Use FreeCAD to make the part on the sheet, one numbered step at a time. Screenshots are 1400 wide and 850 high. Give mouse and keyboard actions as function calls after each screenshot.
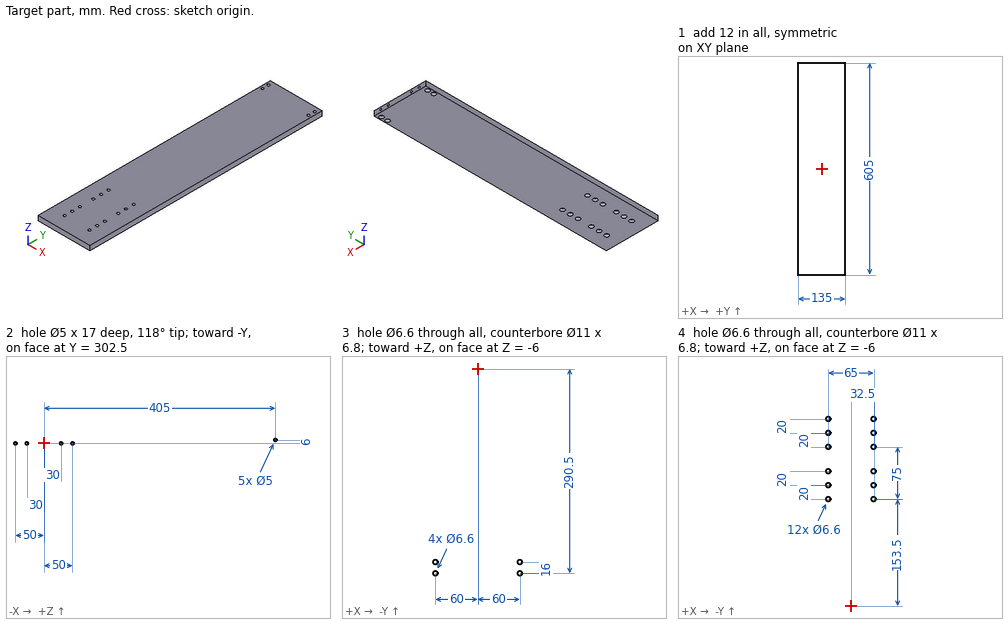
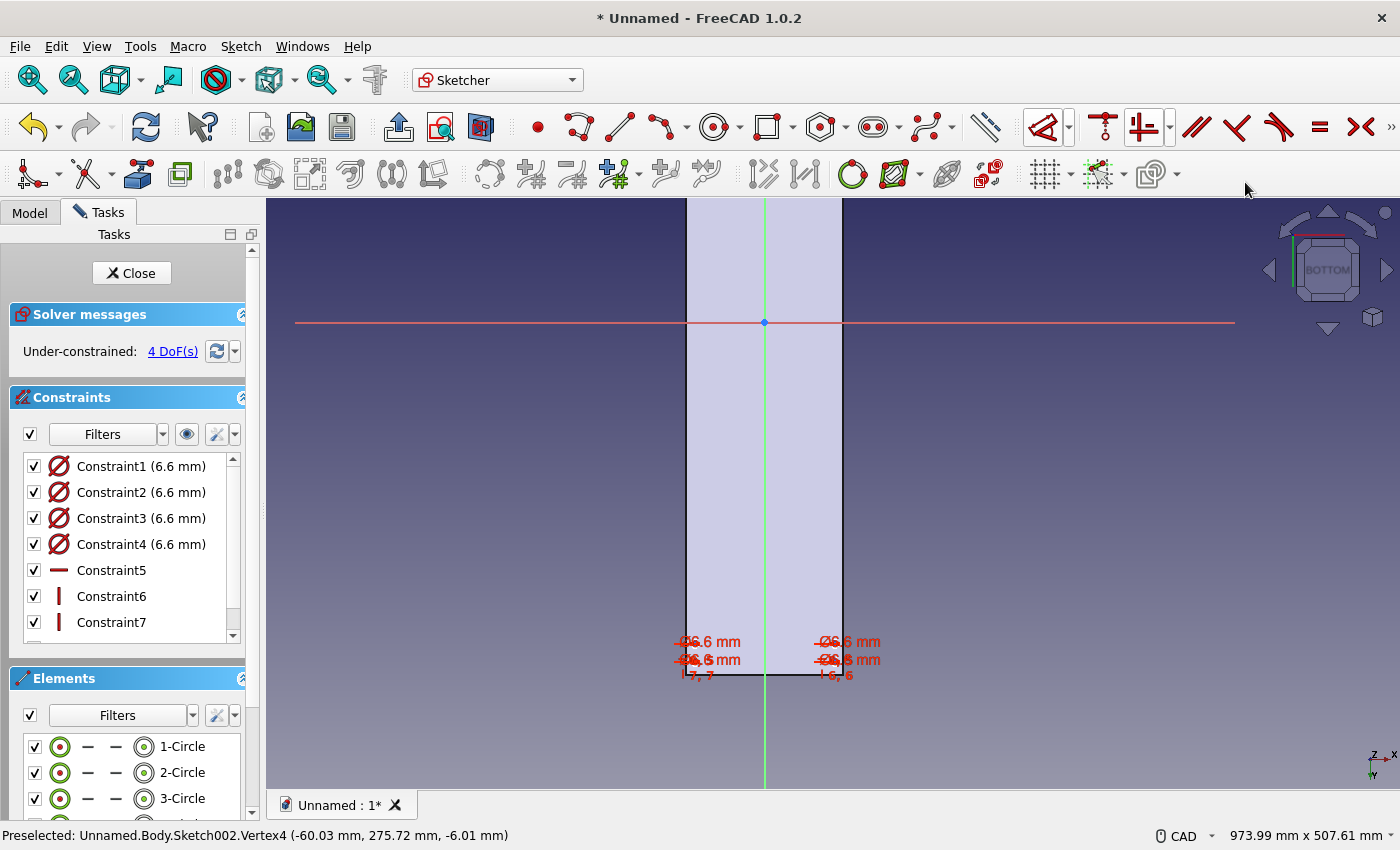
click(835, 662)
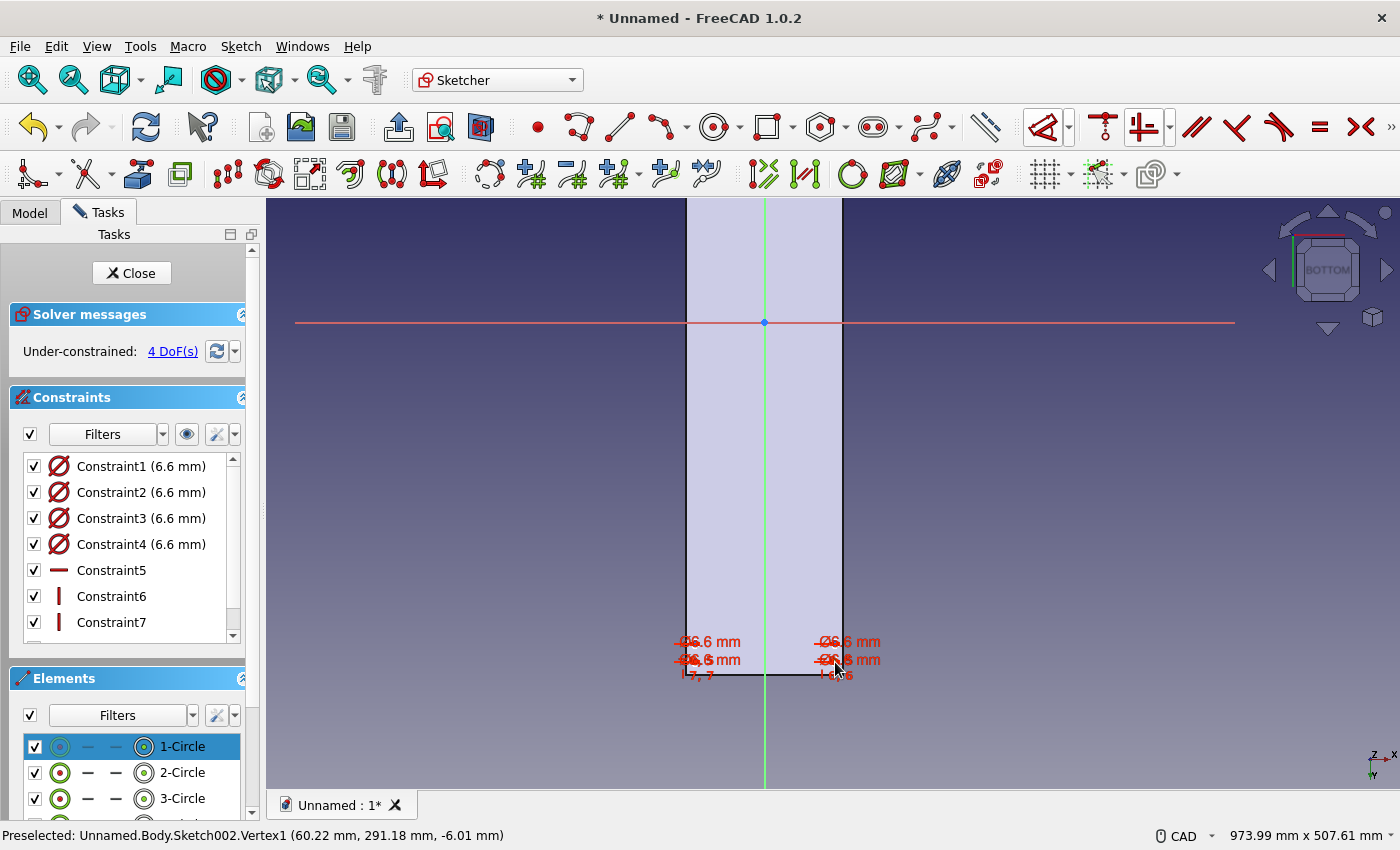
click(1068, 128)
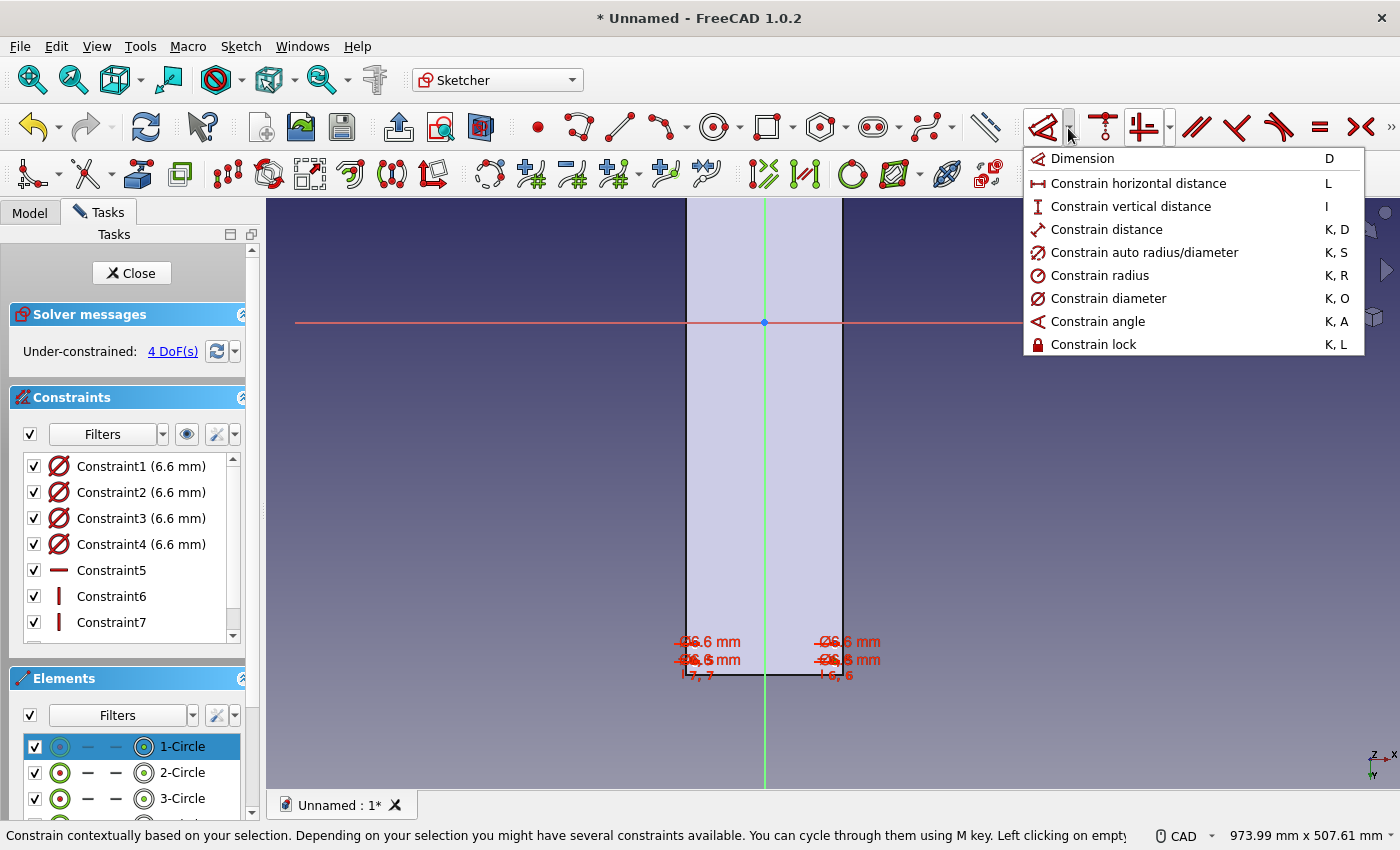
click(1194, 184)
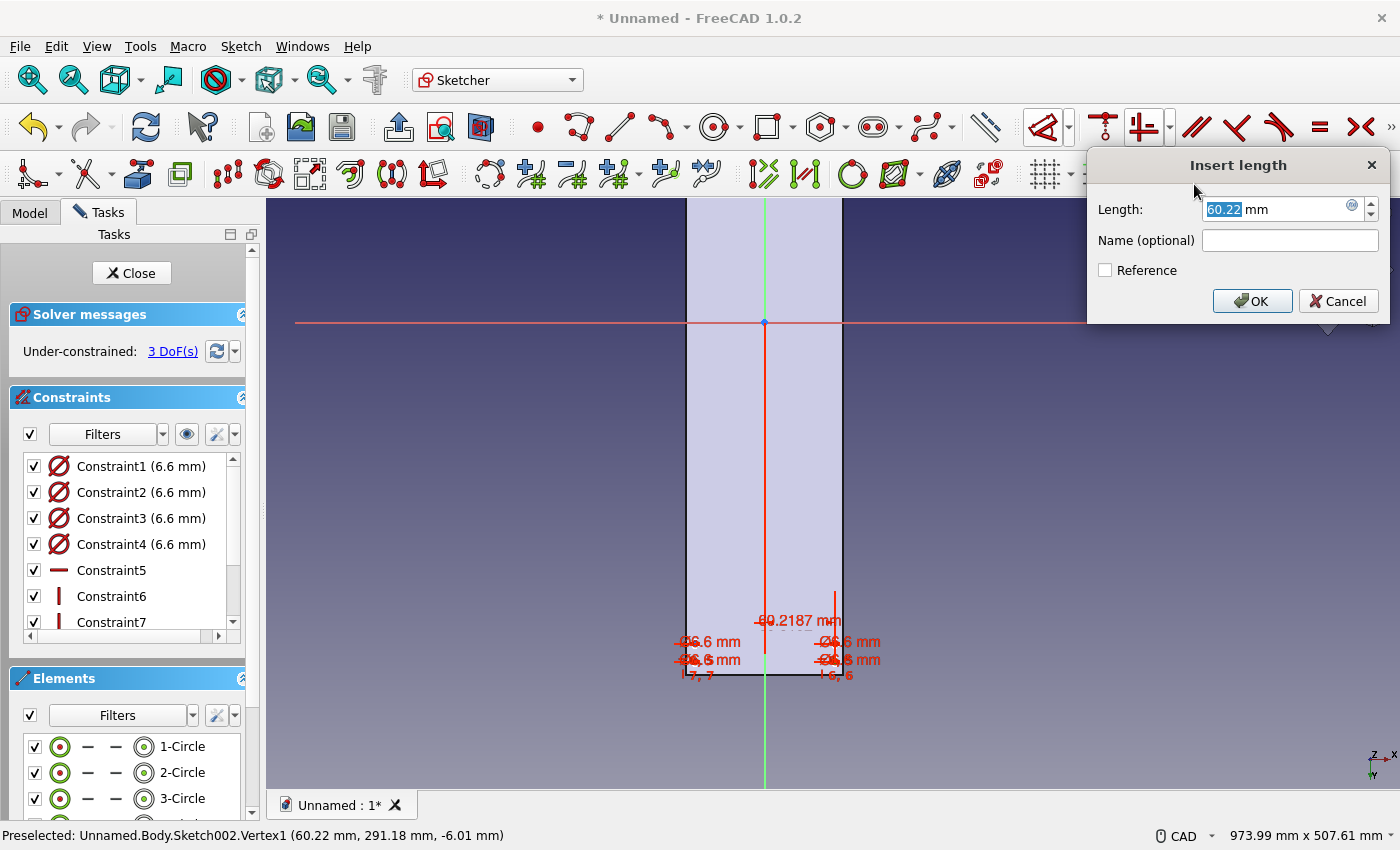
text(60)
key(Return)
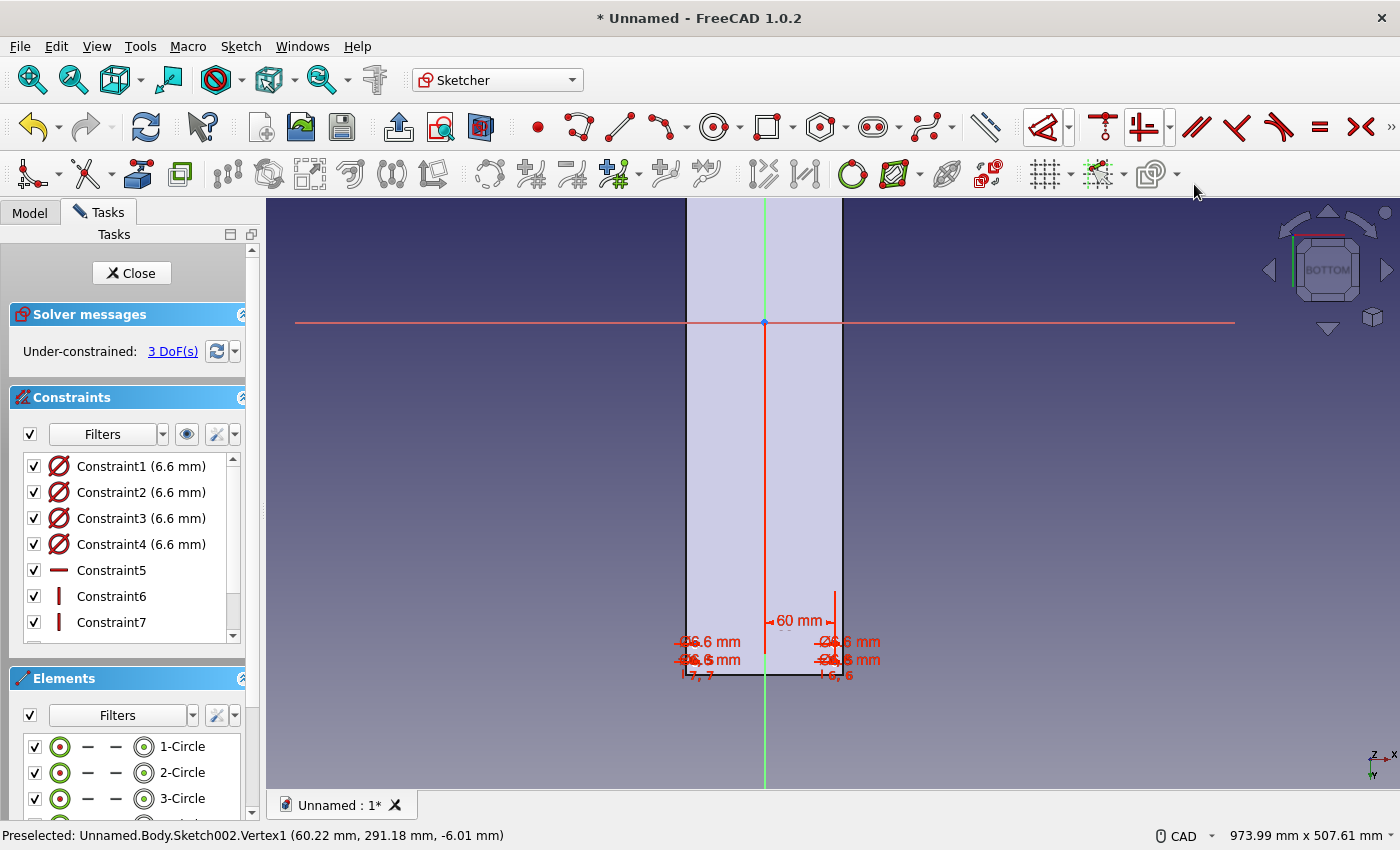
scroll(695, 662, up, 4)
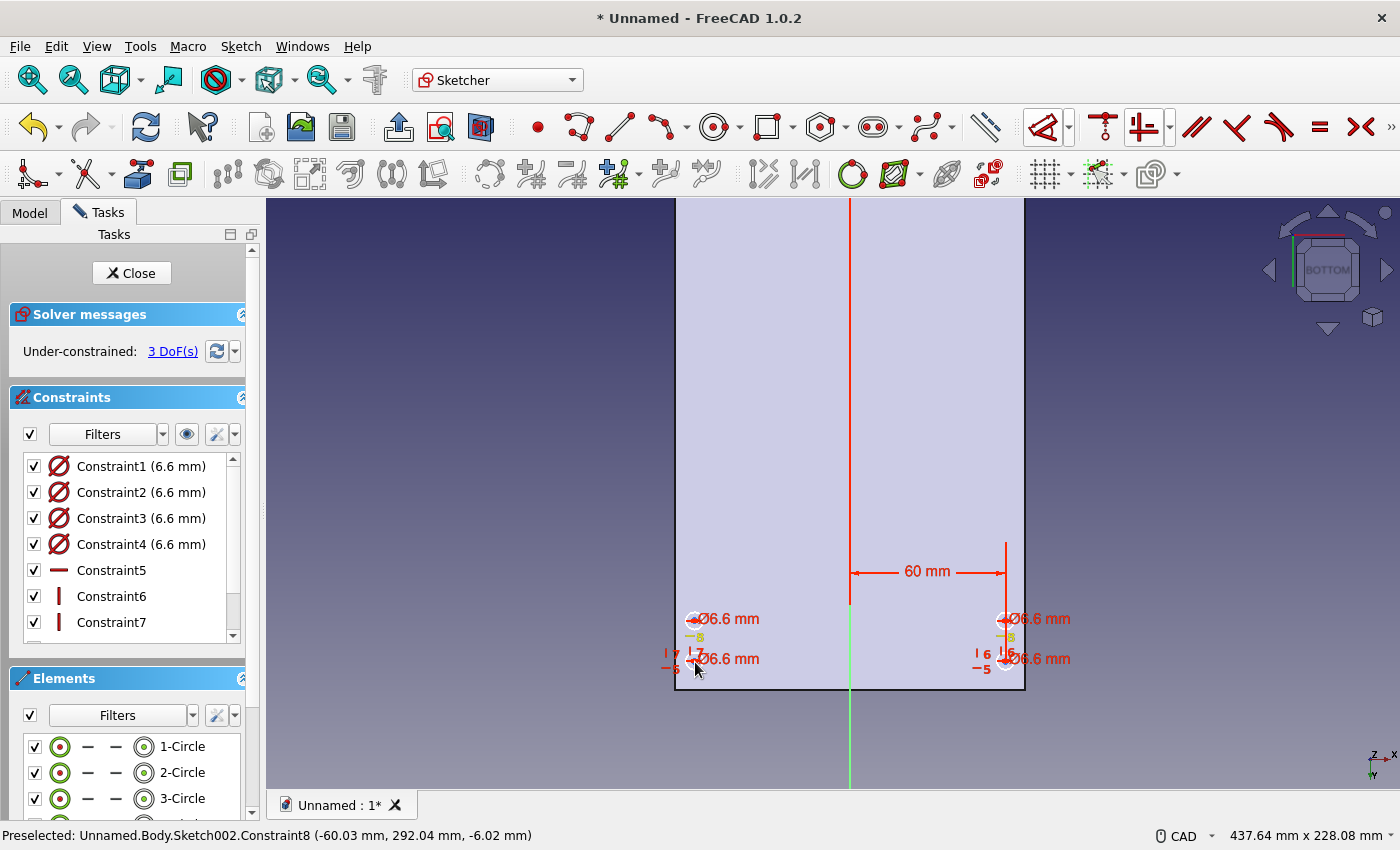
click(695, 661)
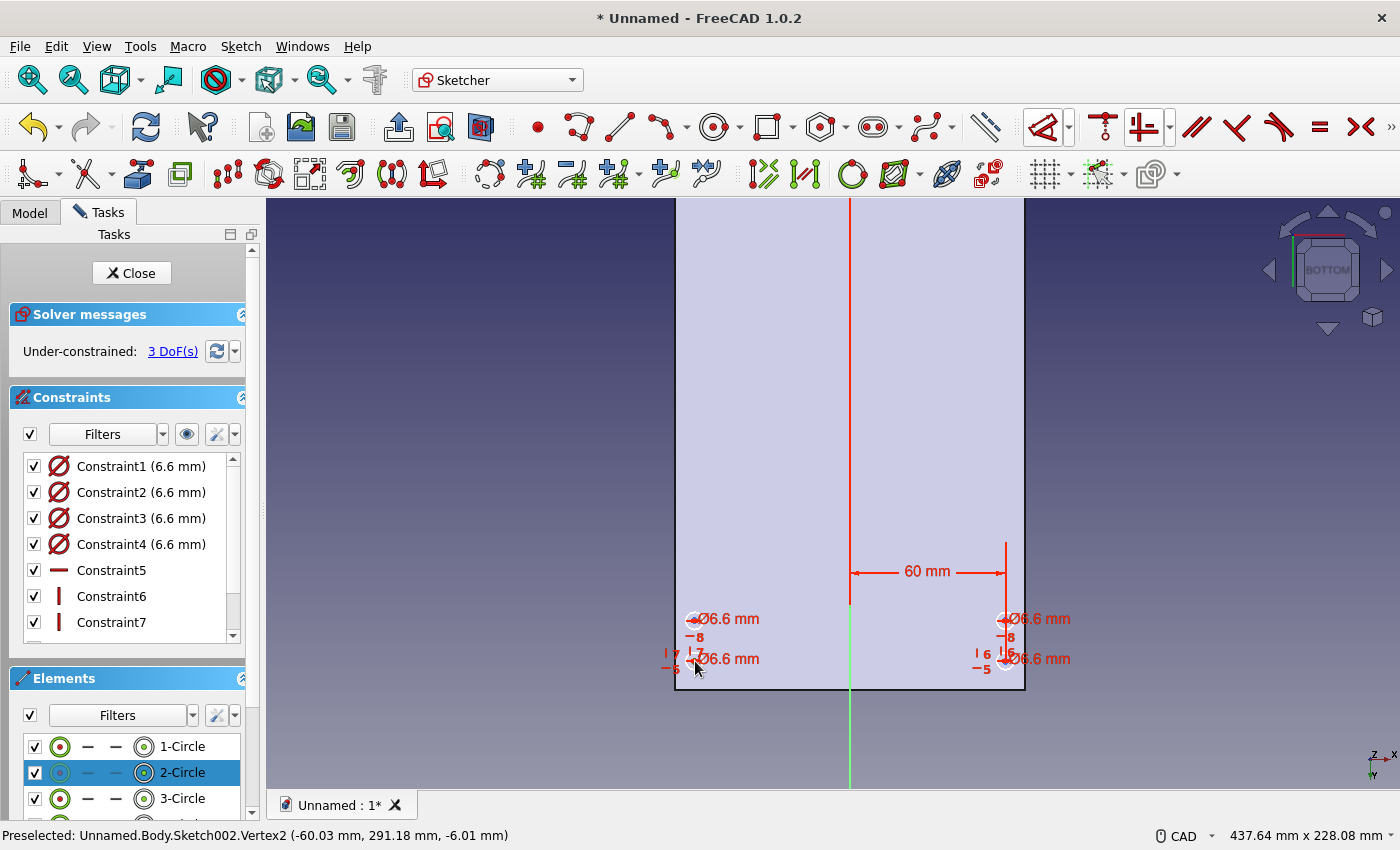
key(l)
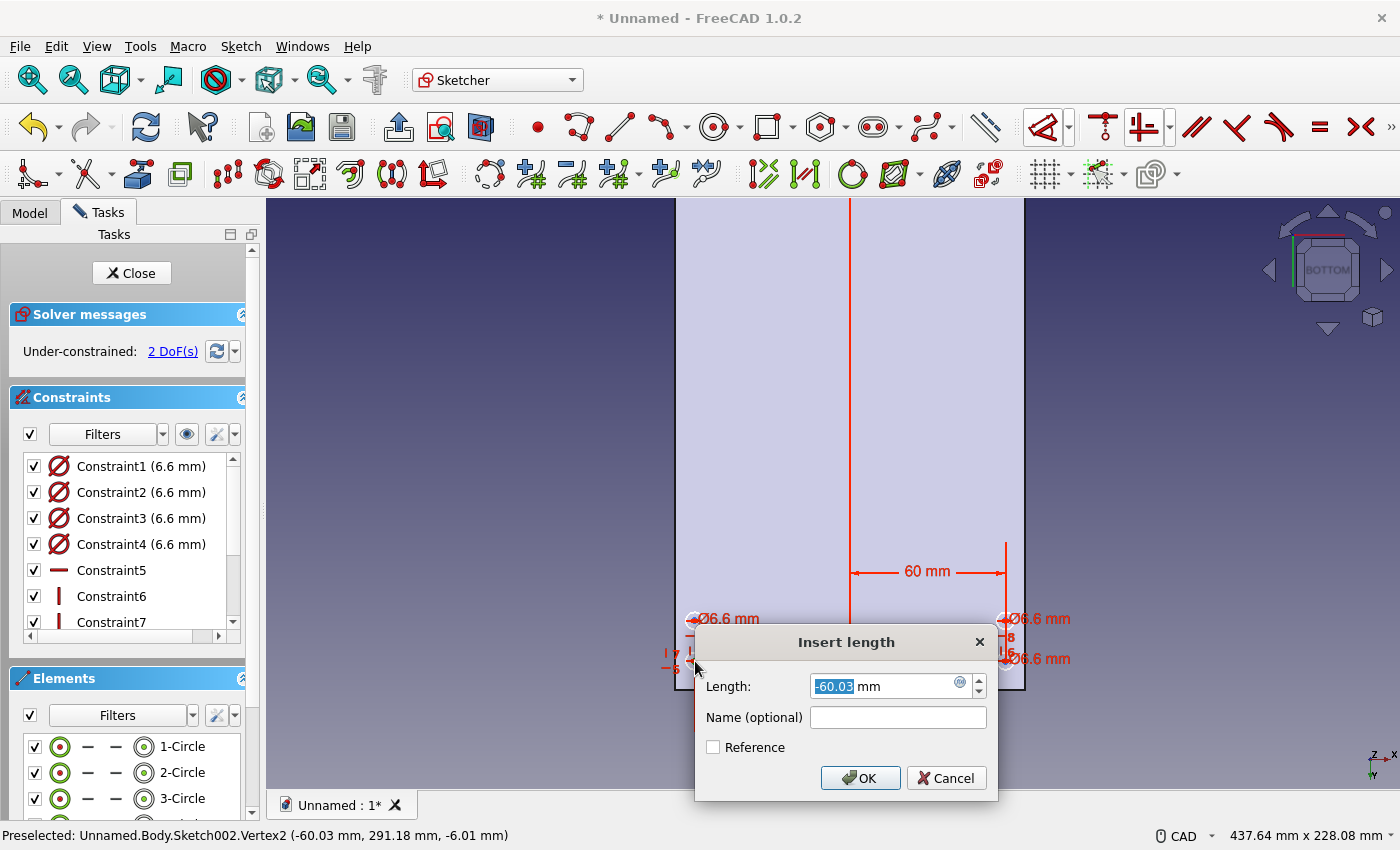
text(-60)
key(Return)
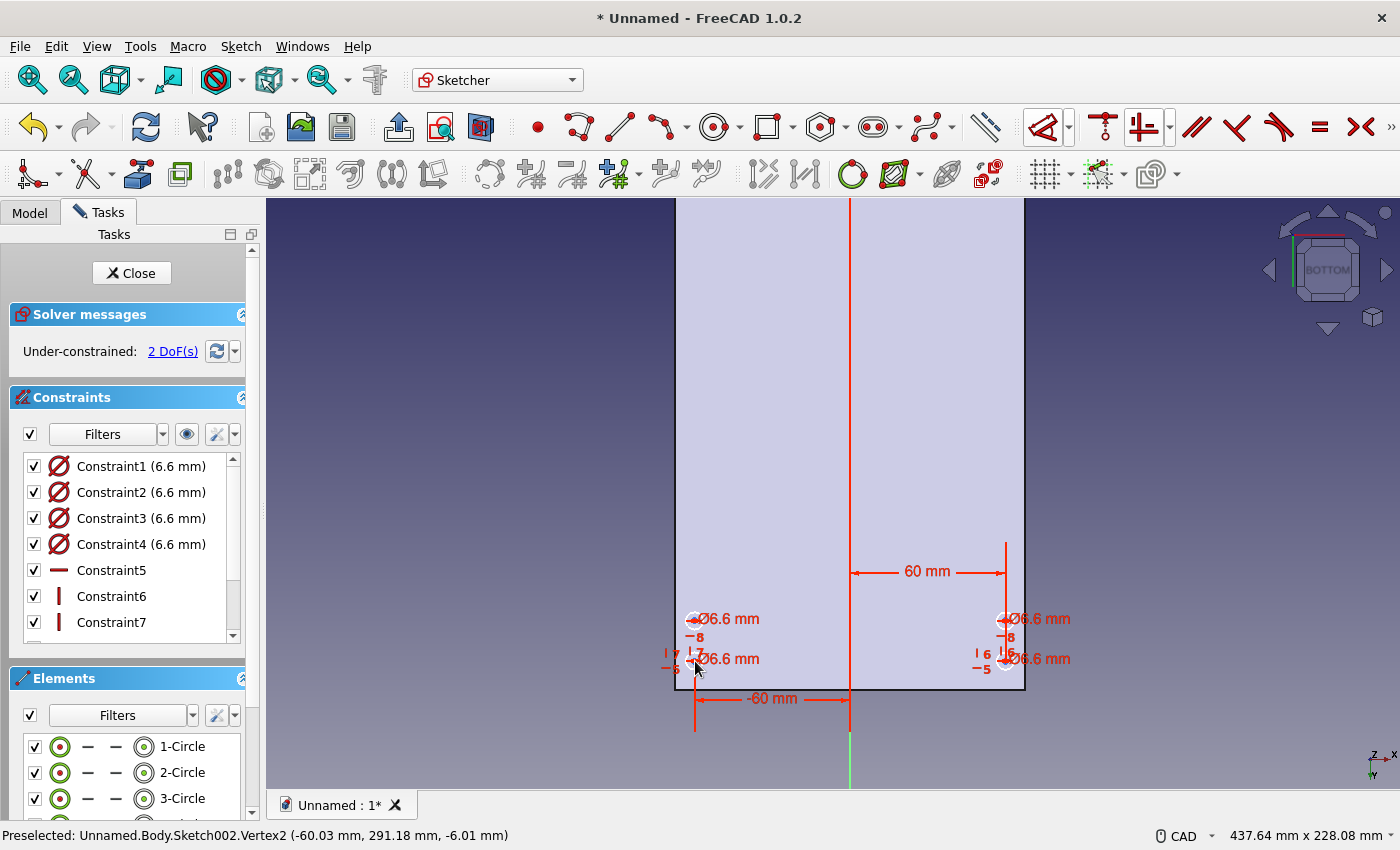
click(1006, 661)